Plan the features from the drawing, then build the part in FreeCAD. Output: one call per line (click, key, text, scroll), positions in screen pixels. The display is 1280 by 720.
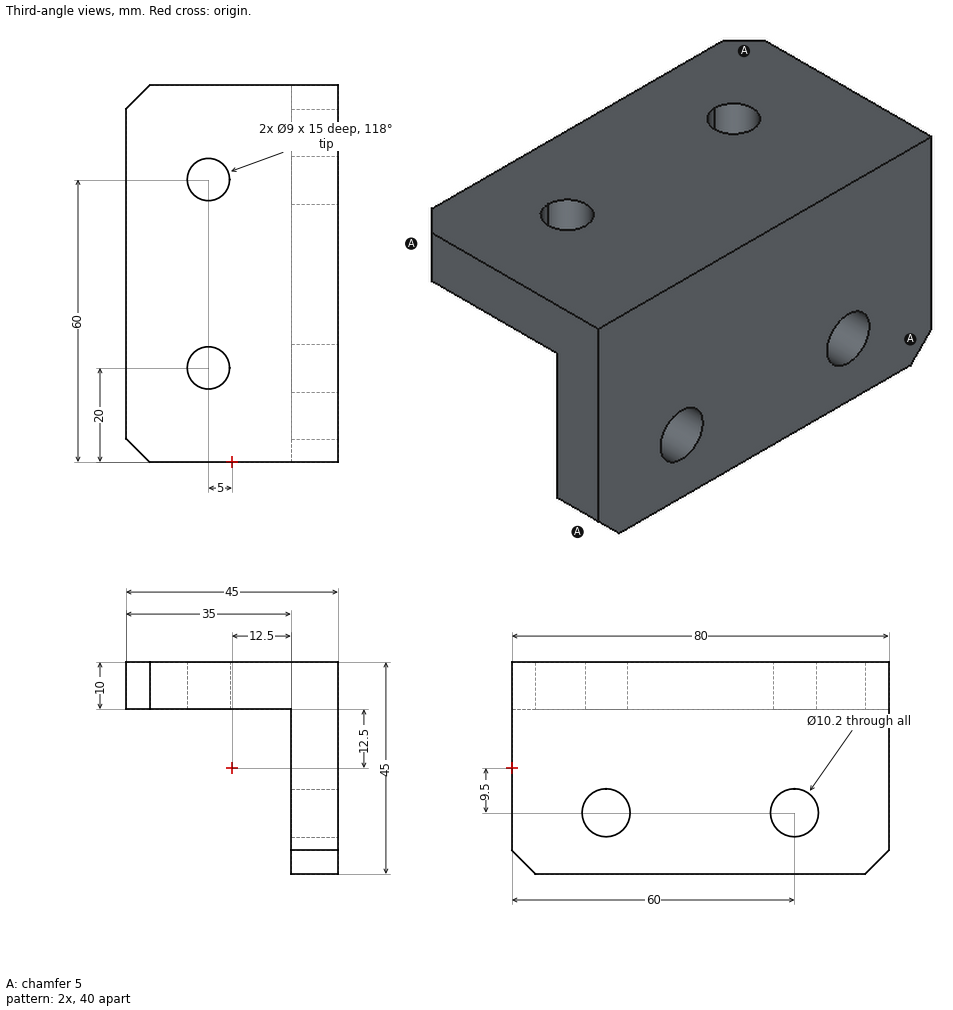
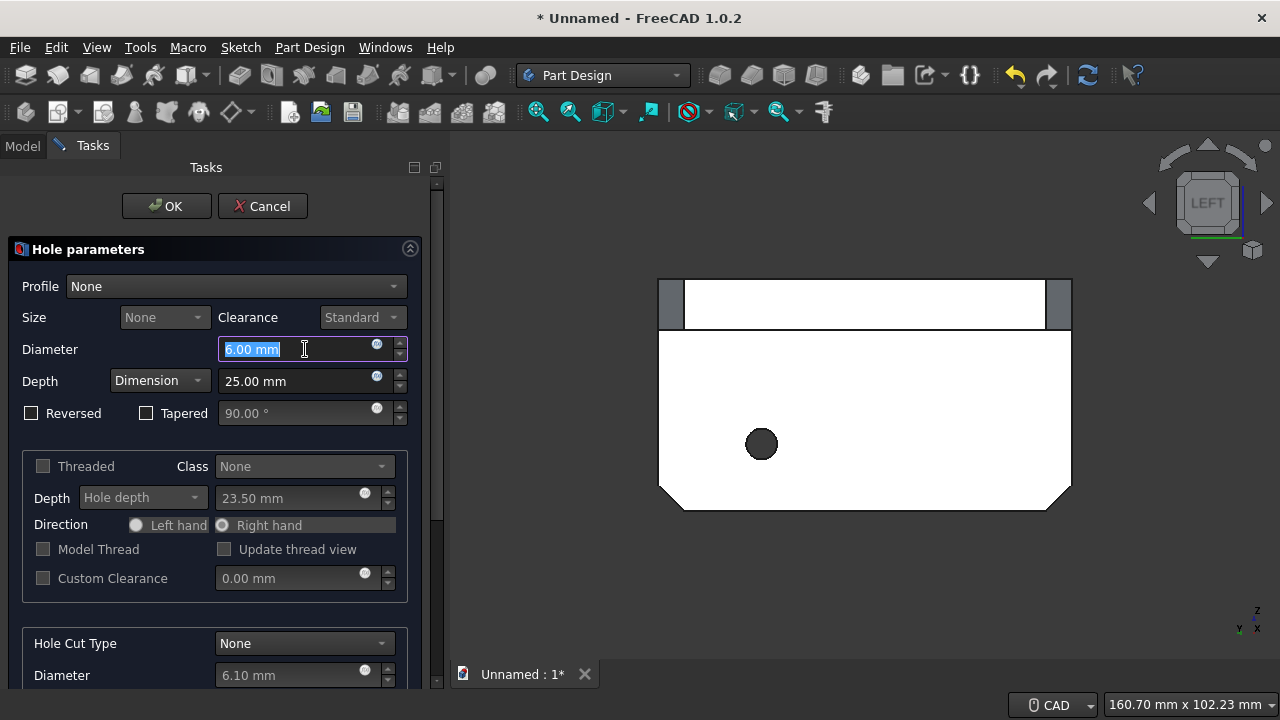
text(10.2)
key(Tab)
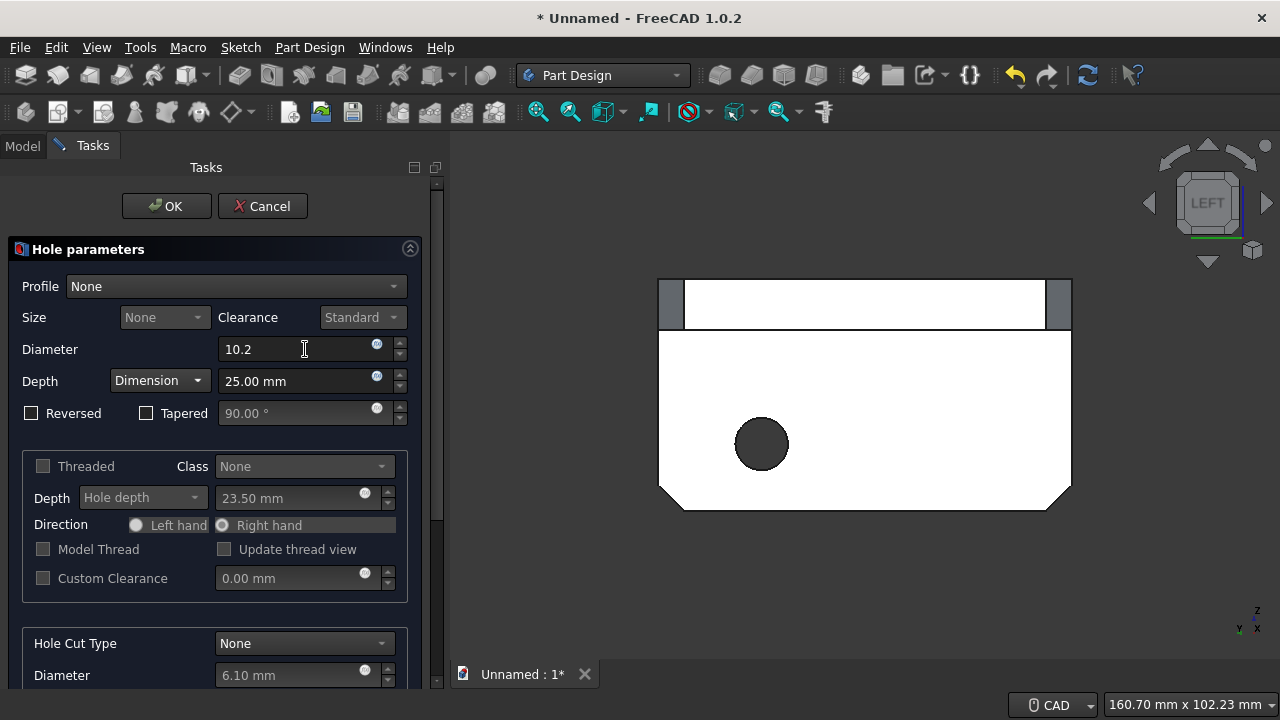
click(161, 380)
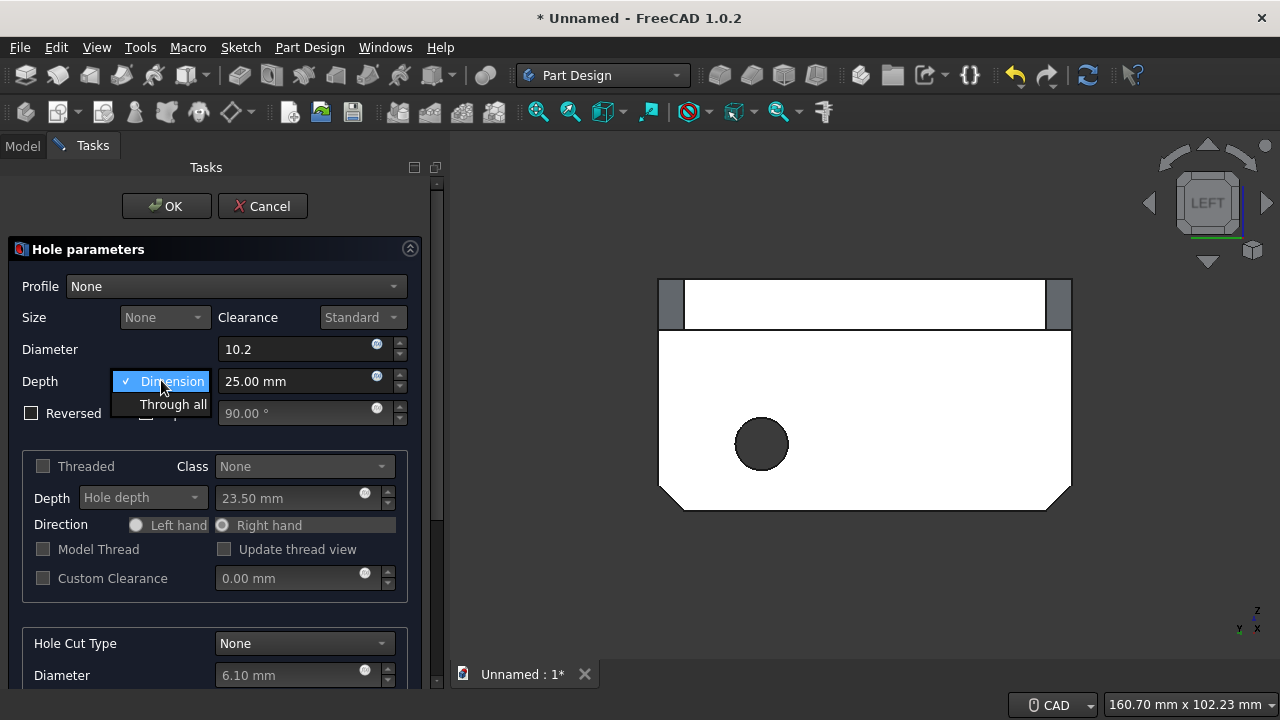
click(160, 404)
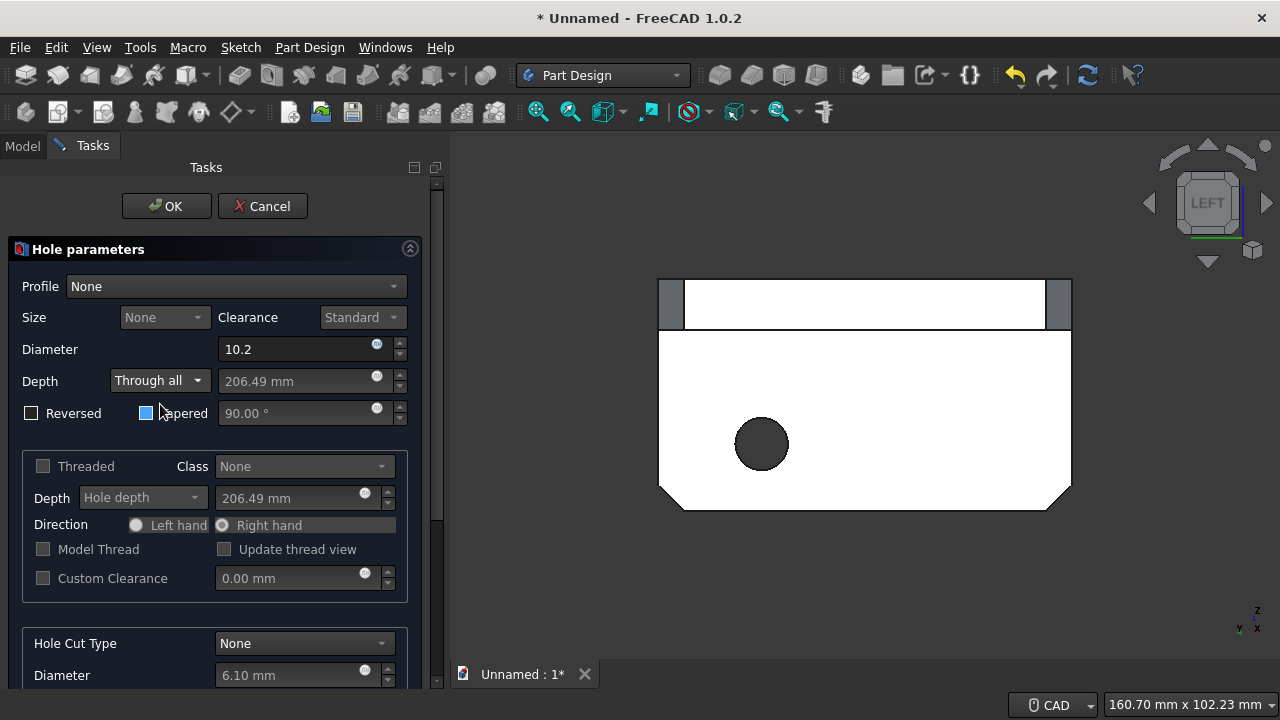
click(167, 206)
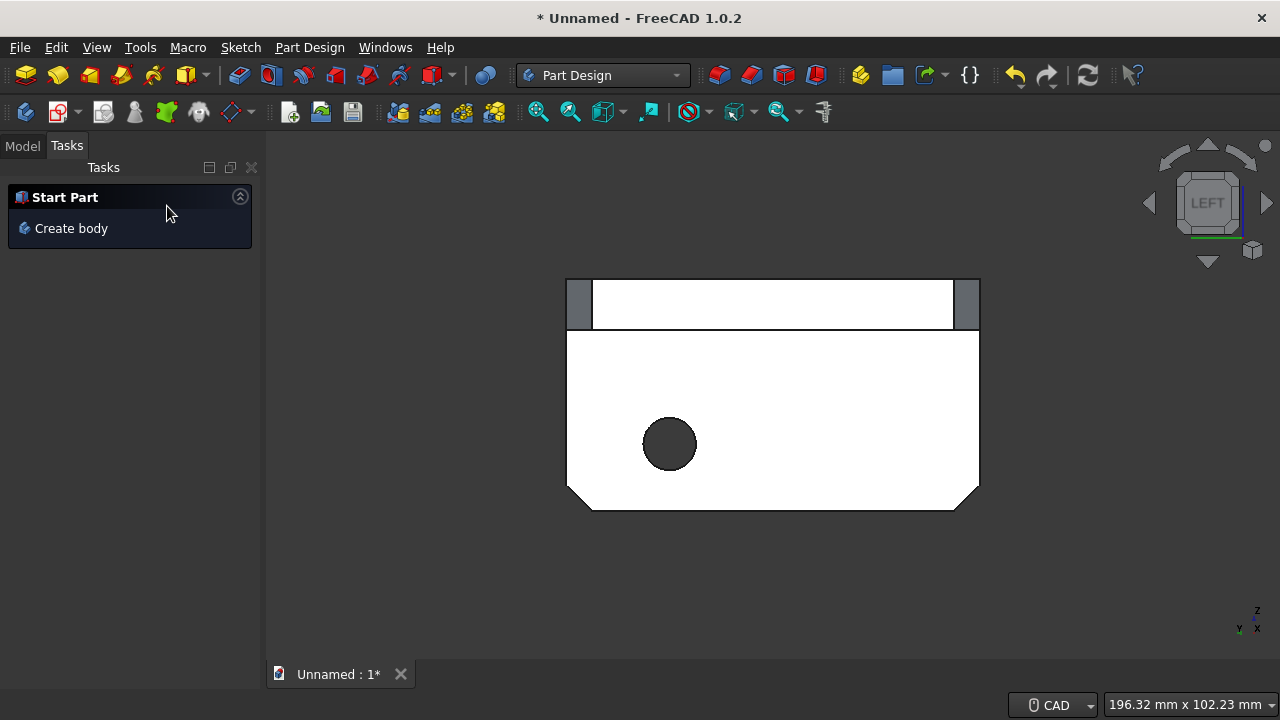
key(v)
key(f)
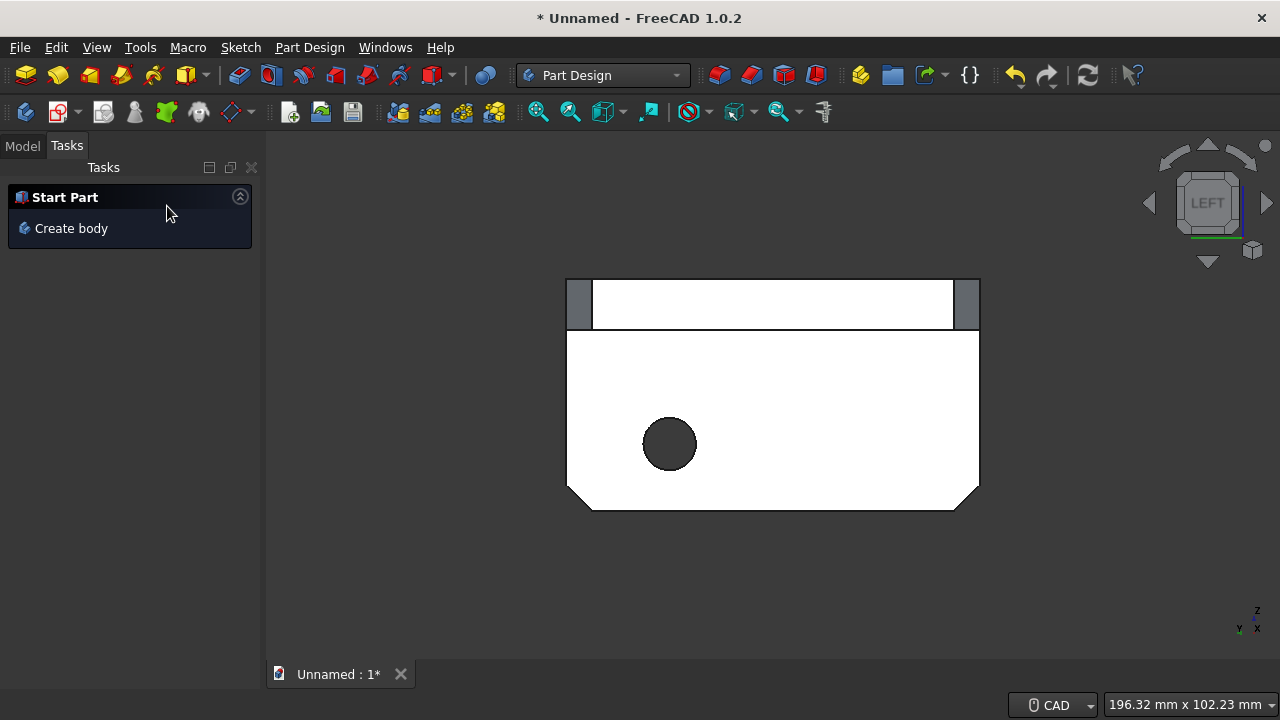
click(23, 145)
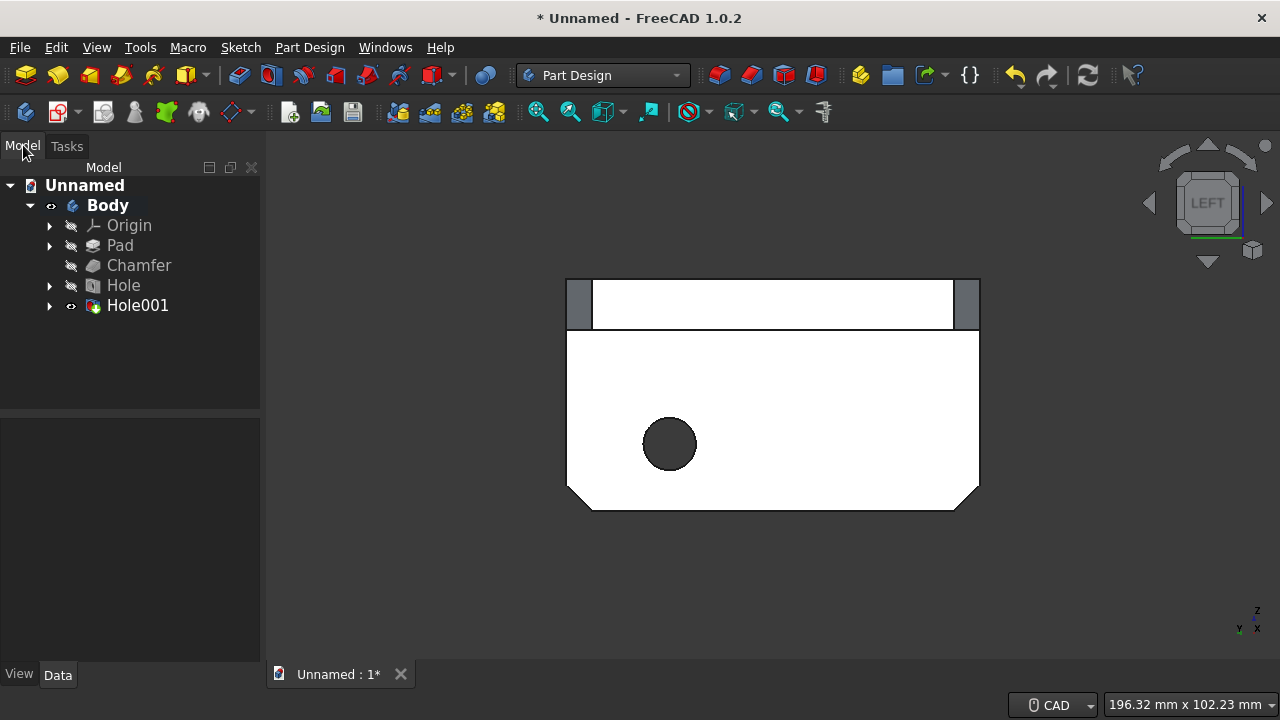
click(116, 306)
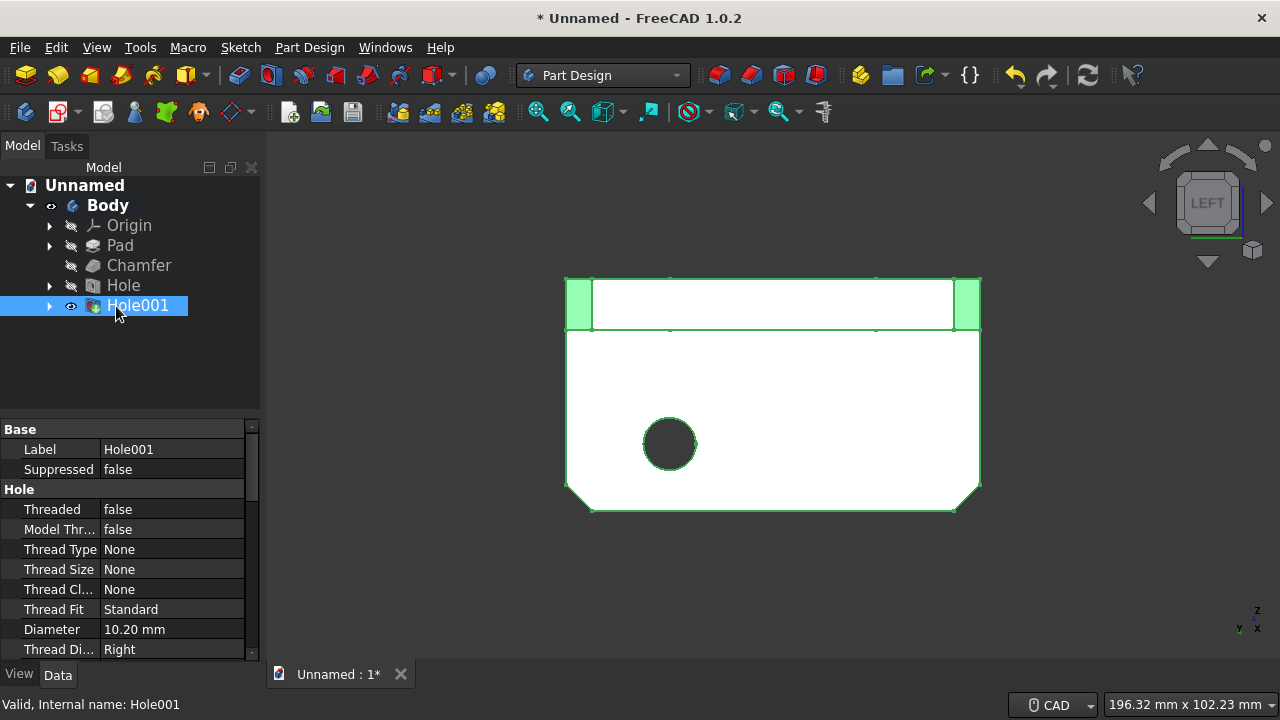
click(430, 112)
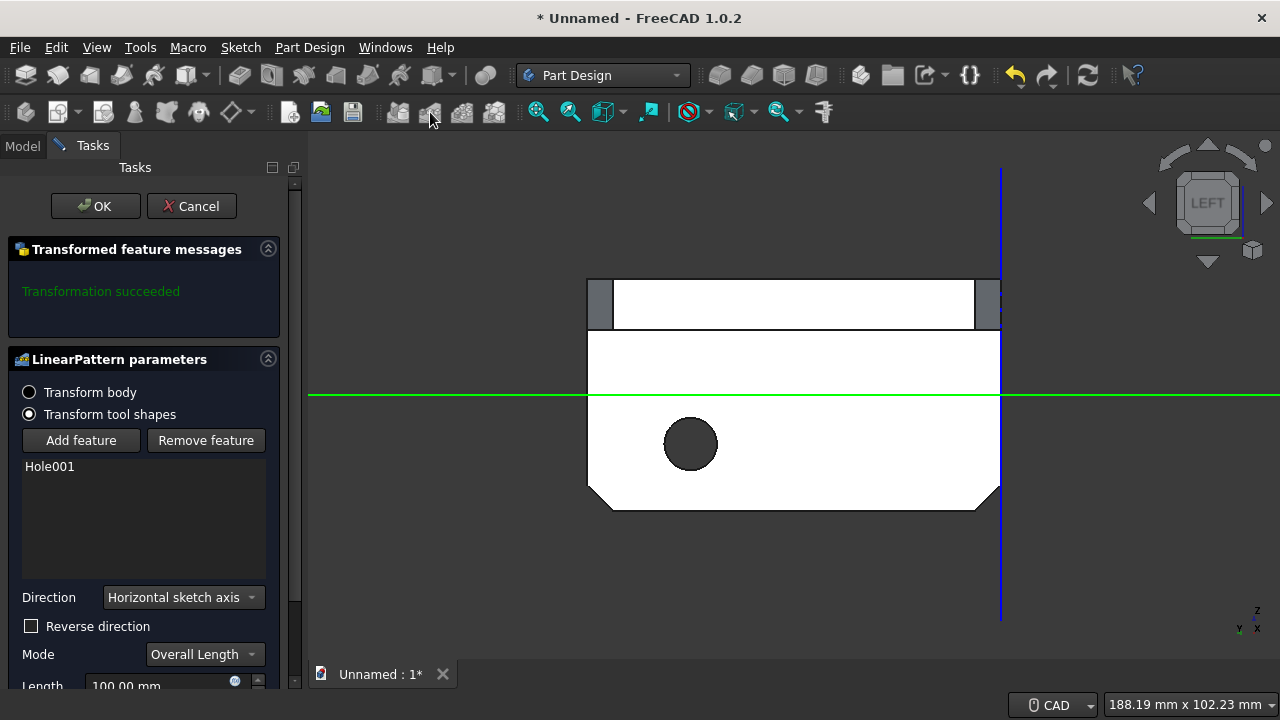
click(184, 598)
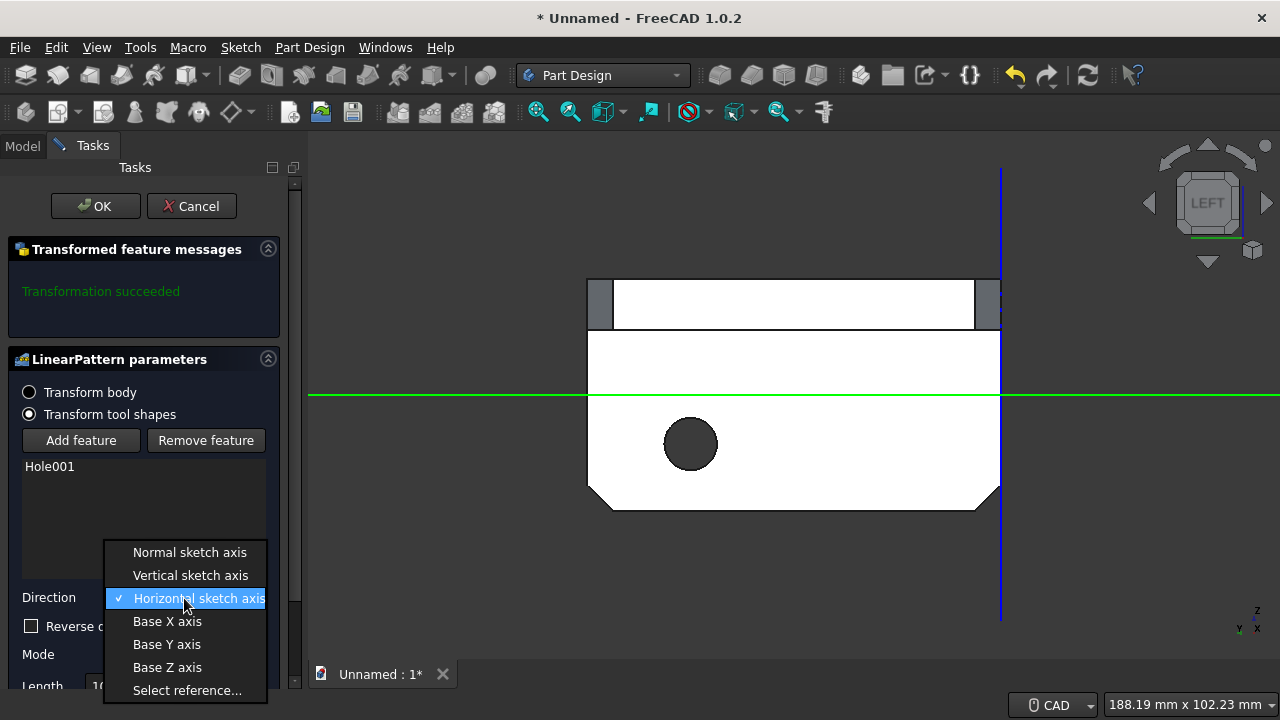
click(184, 644)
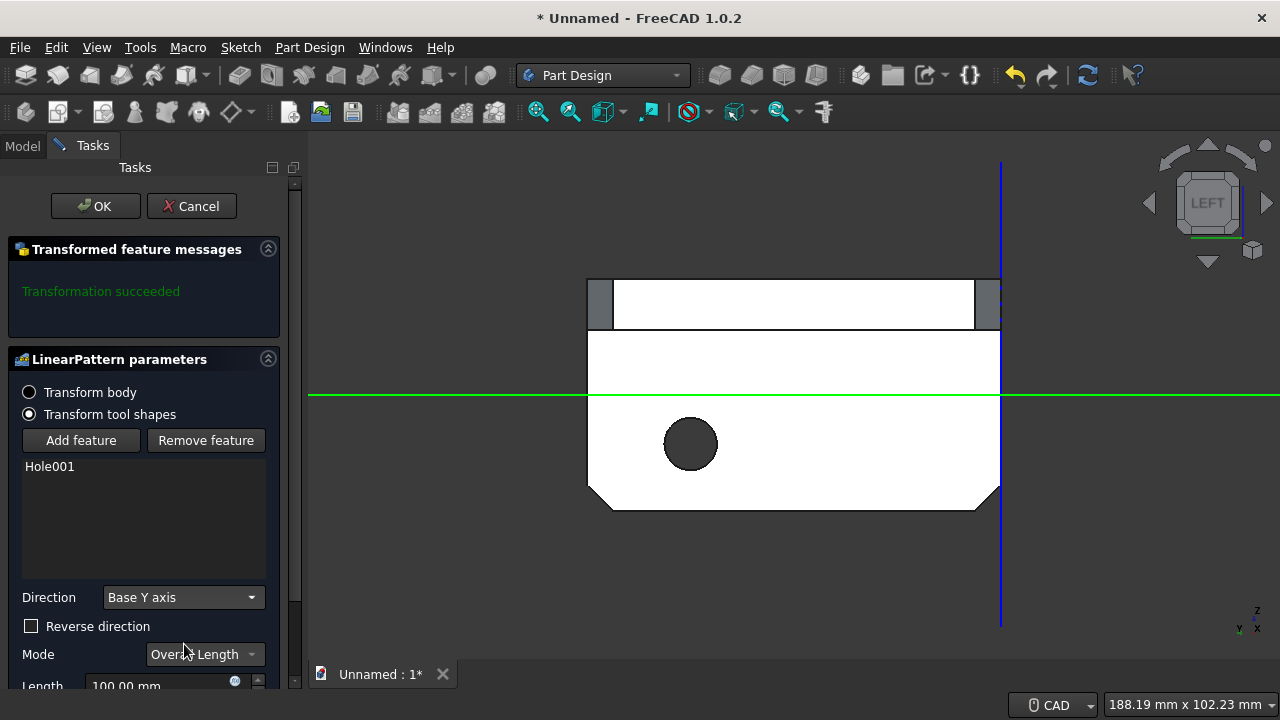
click(206, 654)